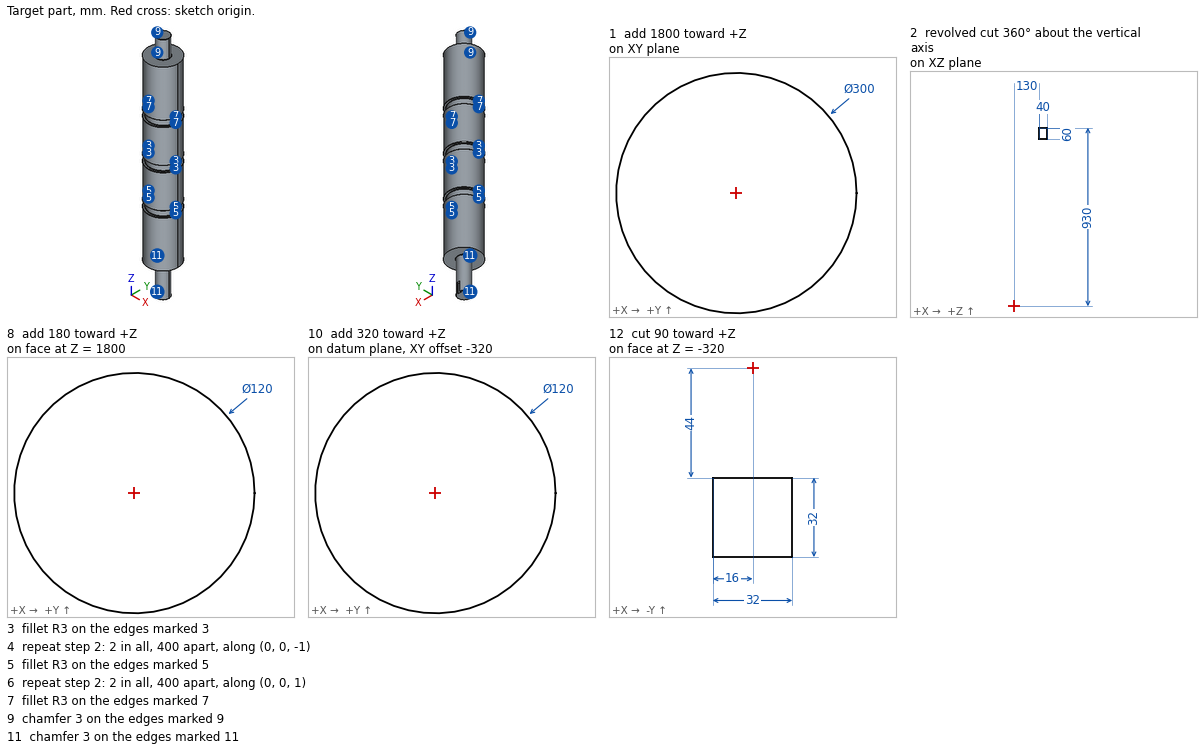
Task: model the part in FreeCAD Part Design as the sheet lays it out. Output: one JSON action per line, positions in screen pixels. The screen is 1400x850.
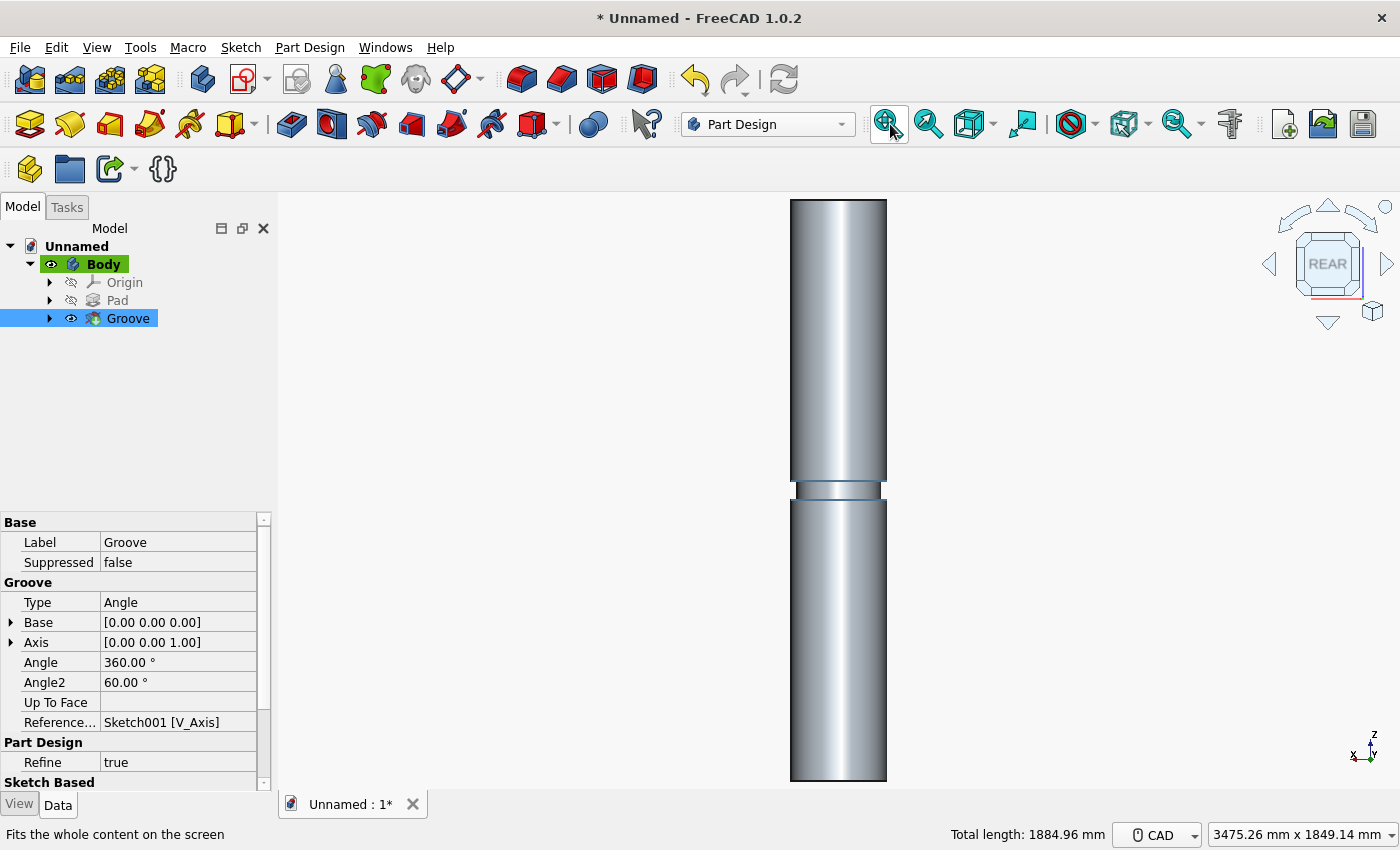
{"action": "key", "text": "6"}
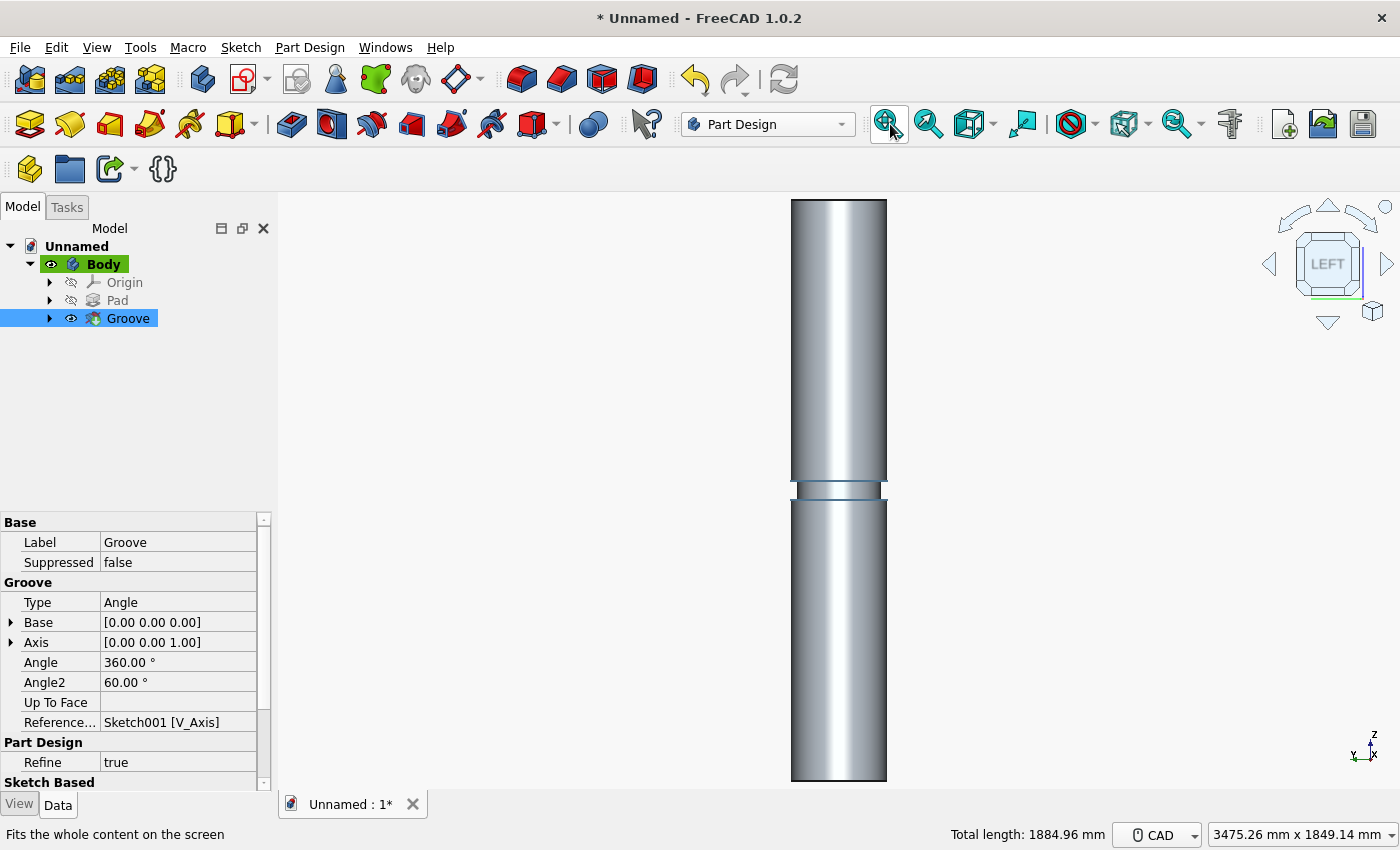
{"action": "key", "text": "v 3"}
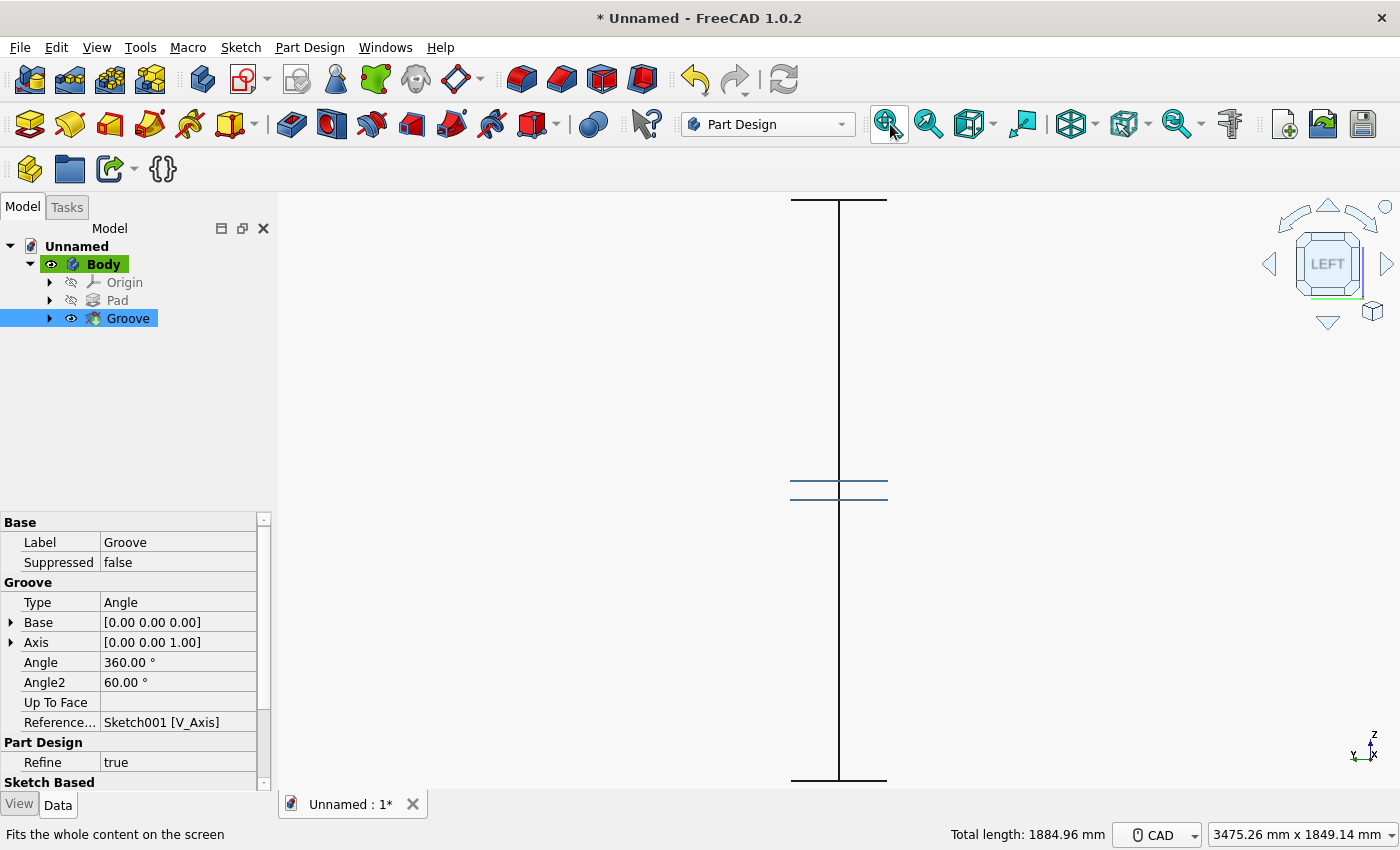
{"action": "key", "text": "0"}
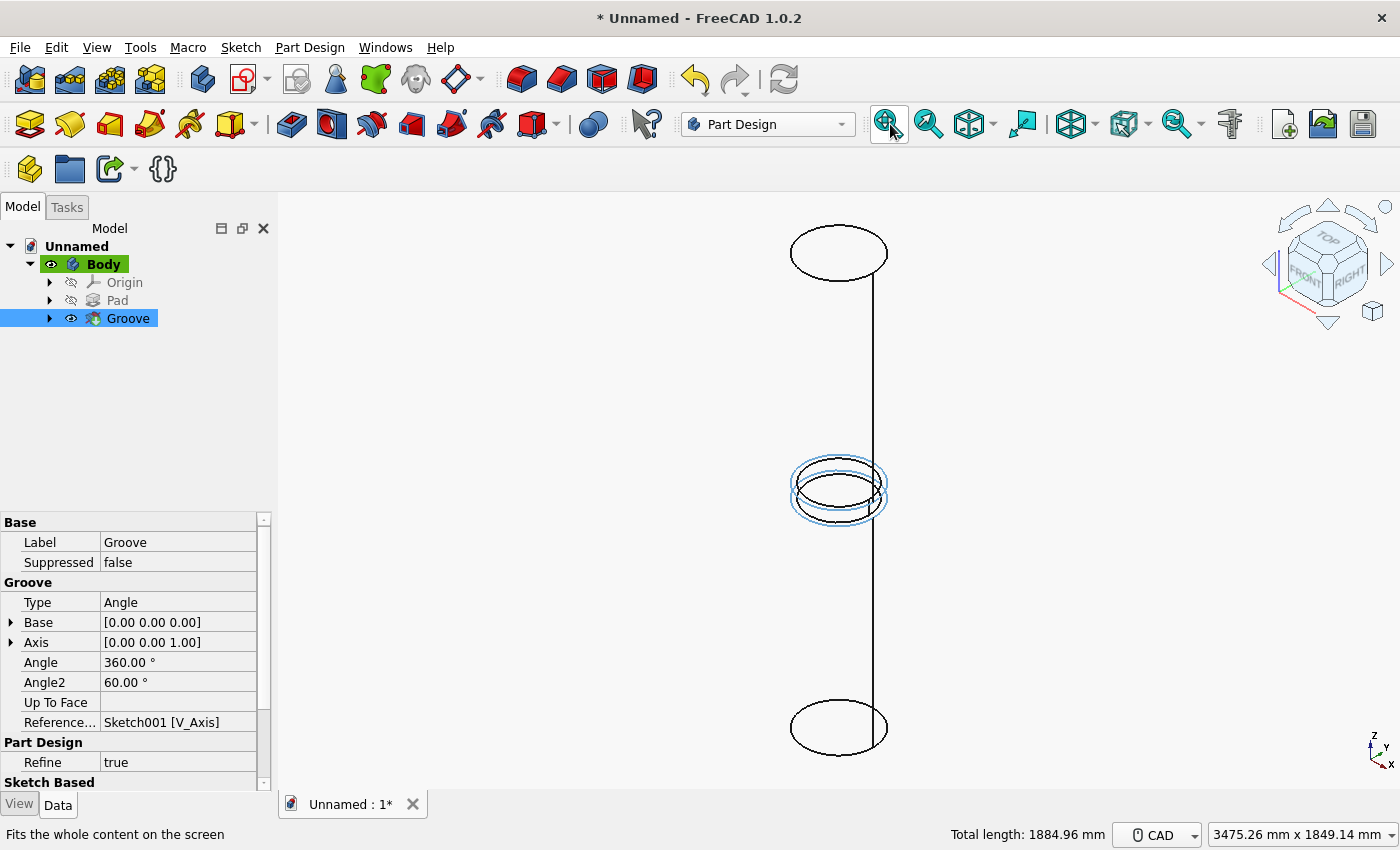
{"action": "left_click", "coordinate": [809, 464], "text": "ctrl"}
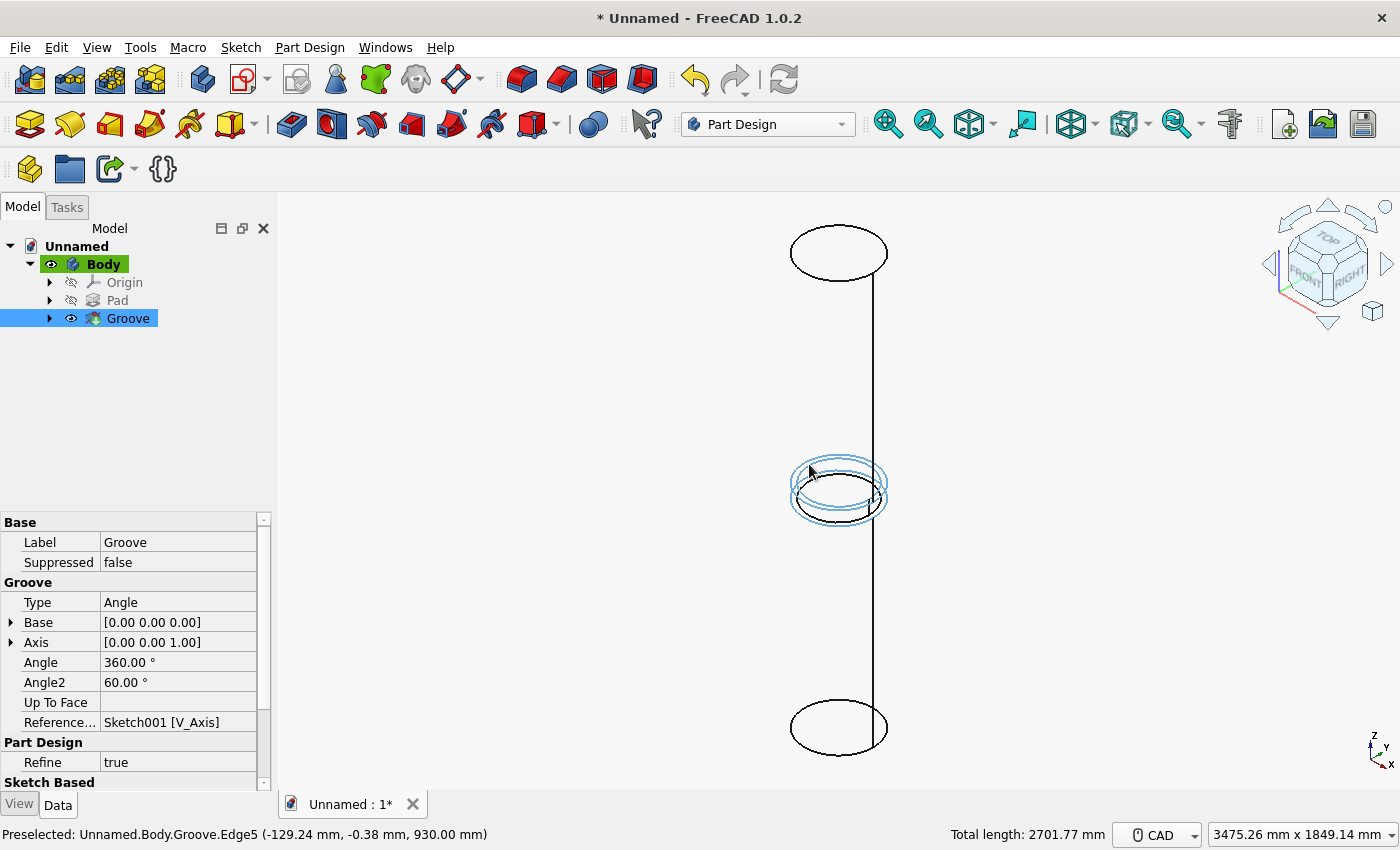
{"action": "left_click", "coordinate": [809, 480], "text": "ctrl"}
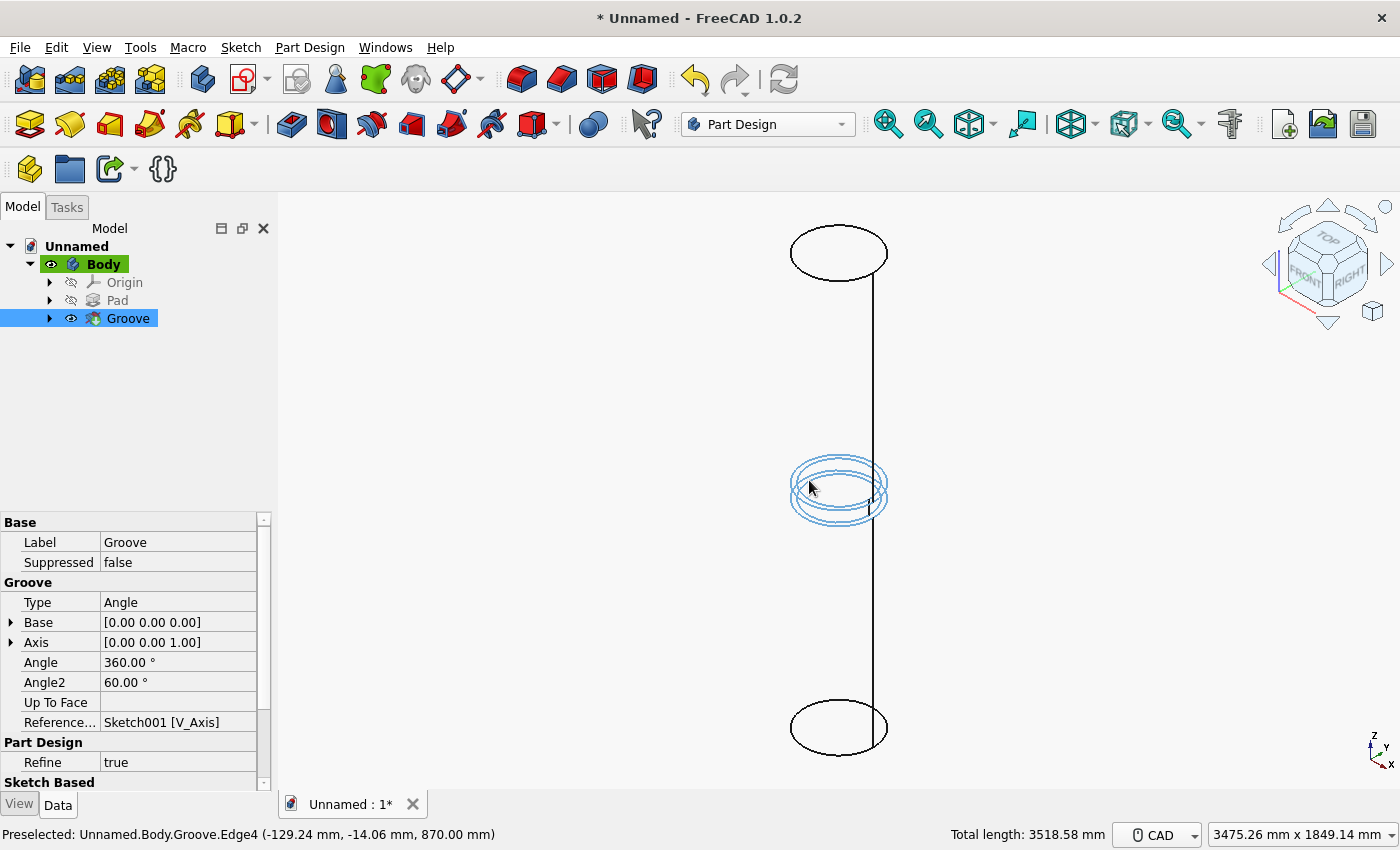
{"action": "key", "text": "v 1"}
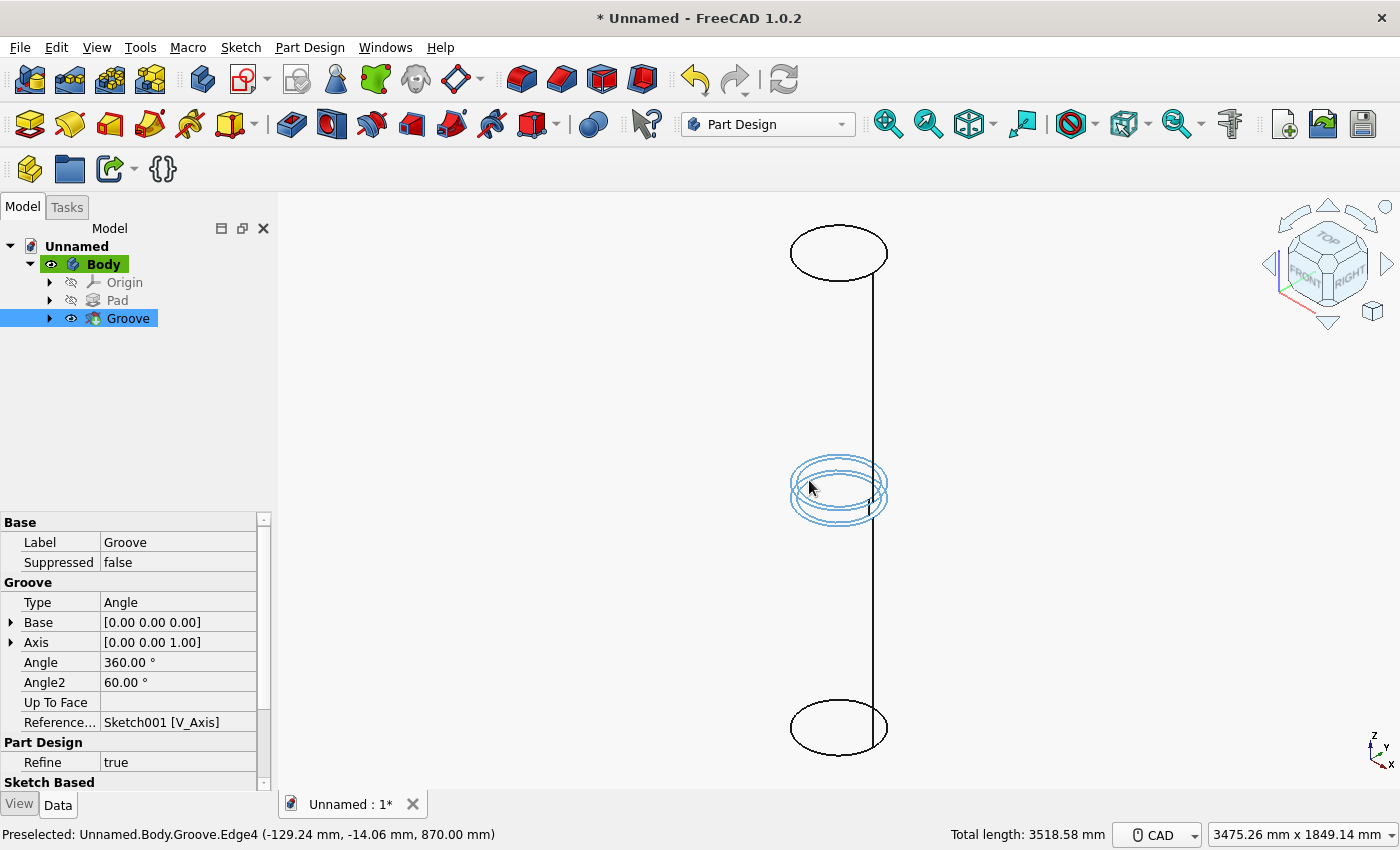
{"action": "left_click", "coordinate": [522, 80]}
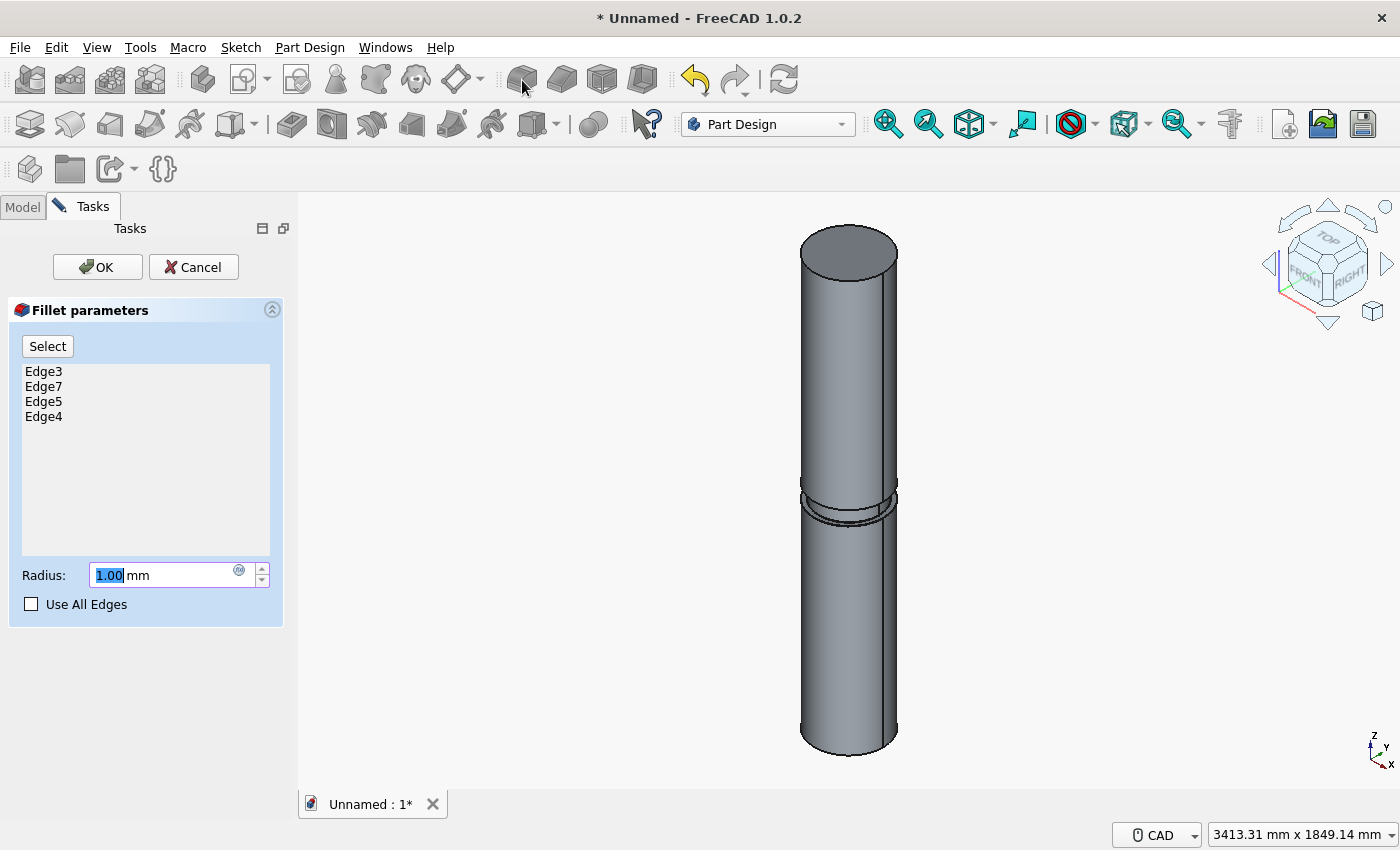
{"action": "type", "text": "3"}
{"action": "key", "text": "Tab"}